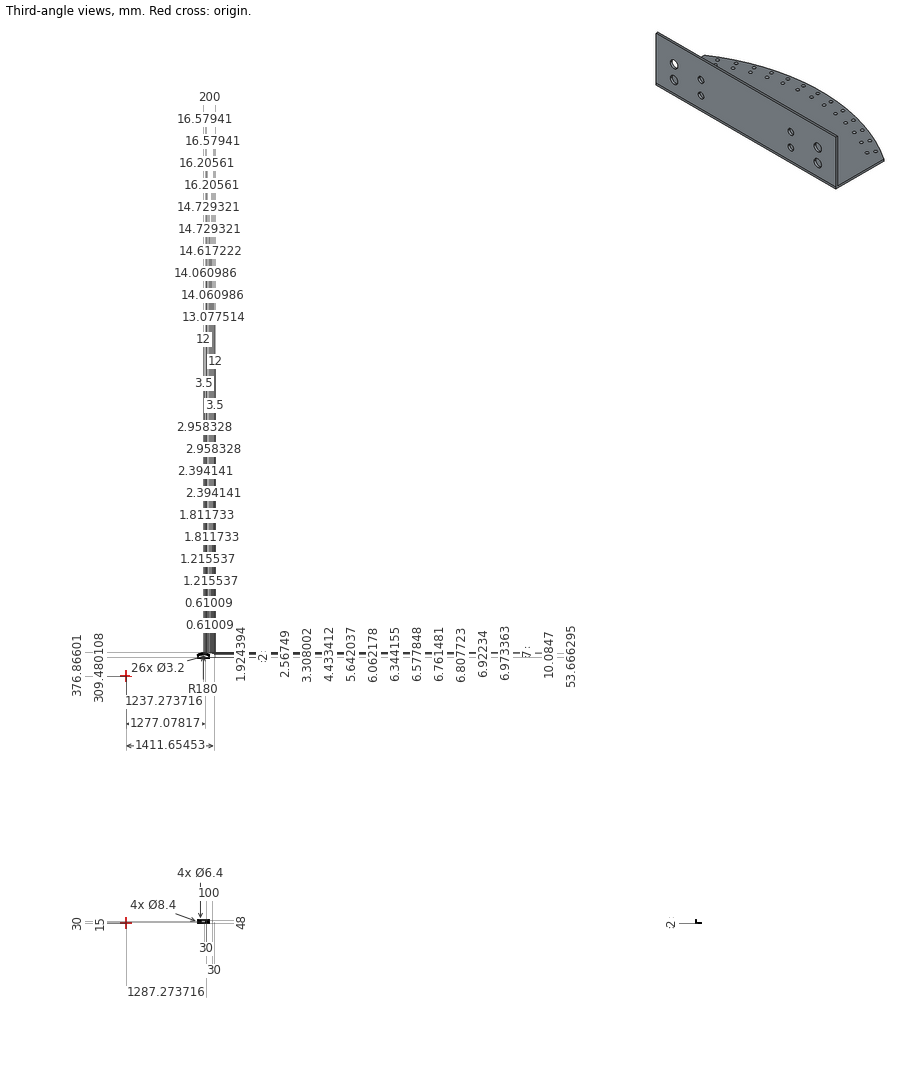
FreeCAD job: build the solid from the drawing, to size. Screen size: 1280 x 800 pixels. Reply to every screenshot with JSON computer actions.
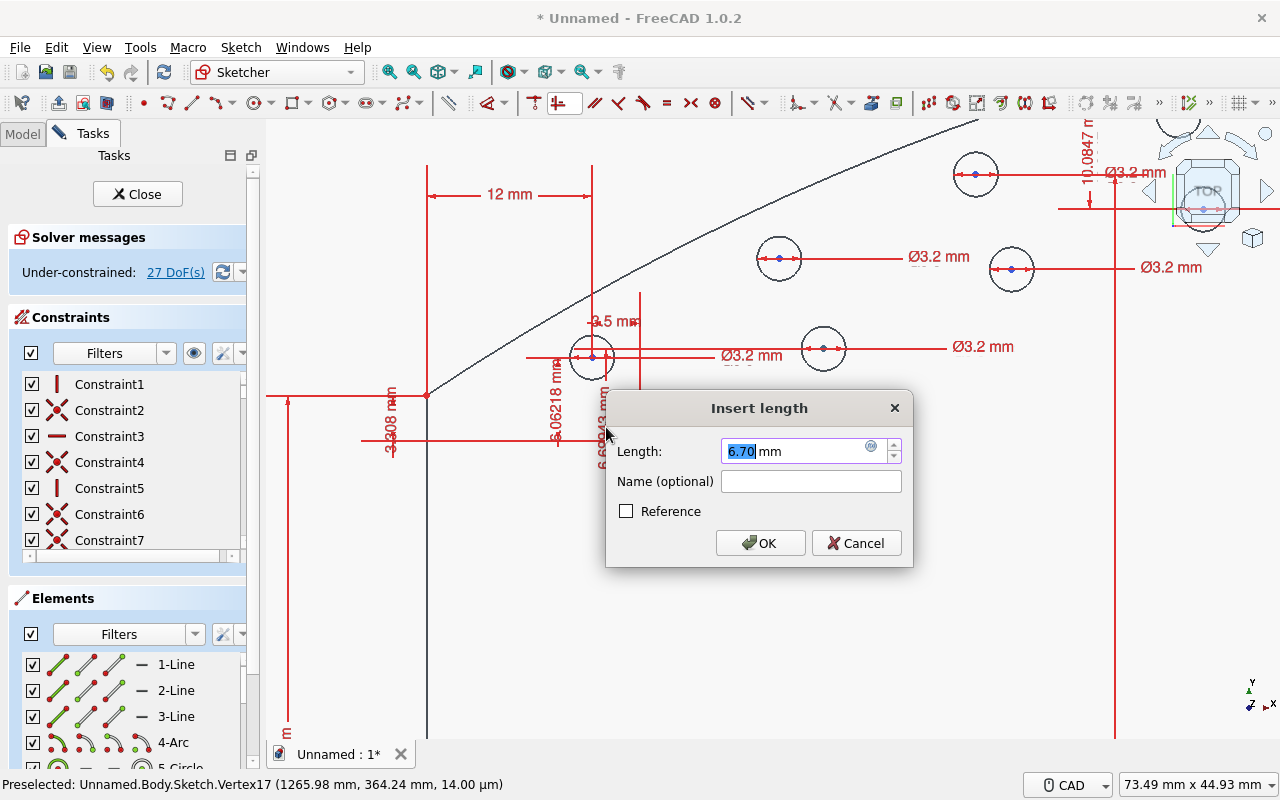
{"action": "type", "text": "6.807723"}
{"action": "key", "text": "Return"}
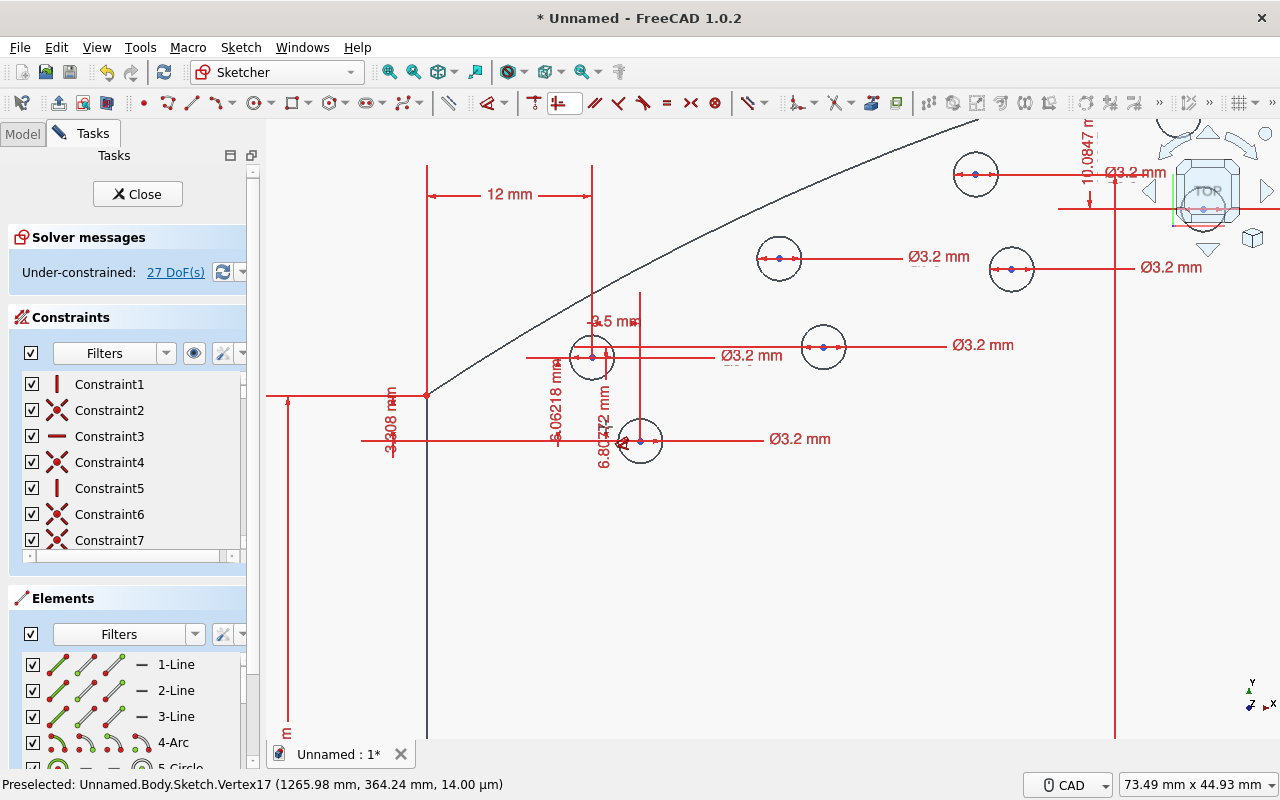
{"action": "left_click", "coordinate": [824, 347]}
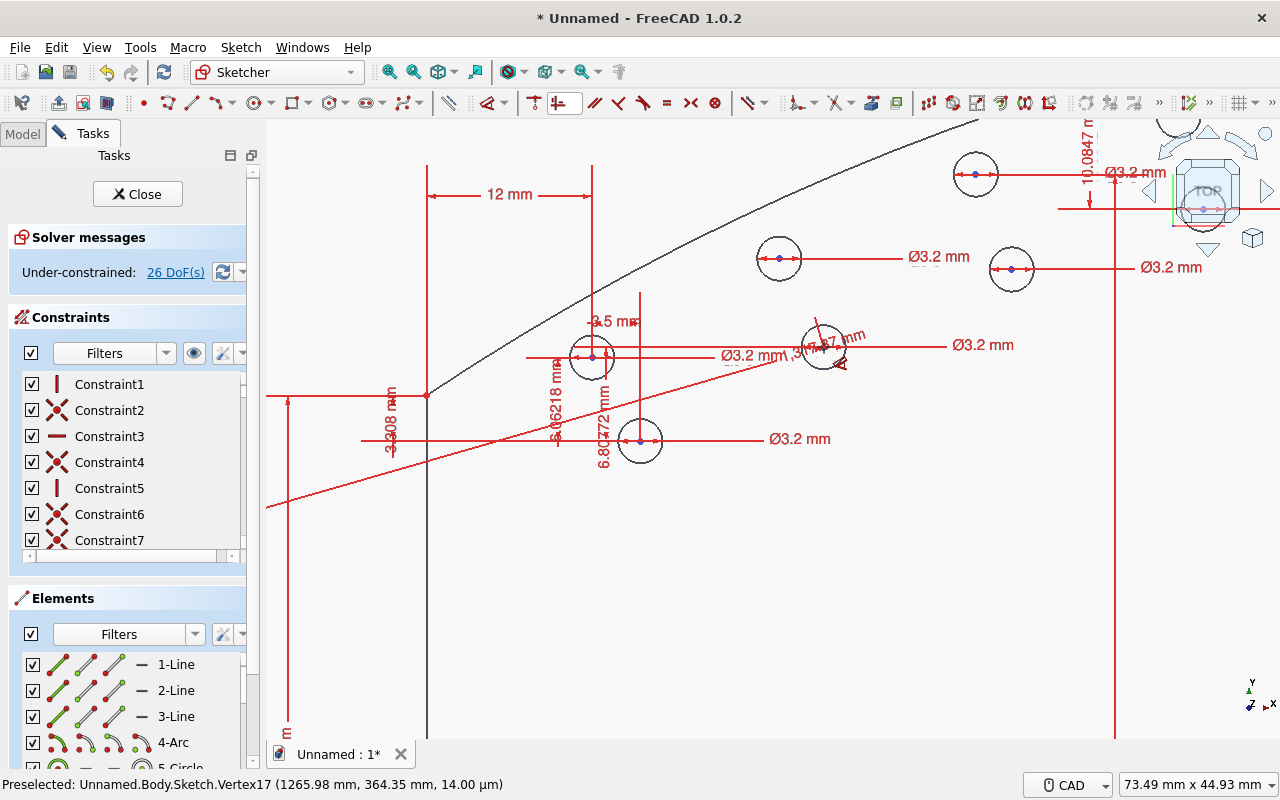
{"action": "left_click", "coordinate": [1012, 269]}
{"action": "left_click", "coordinate": [790, 308]}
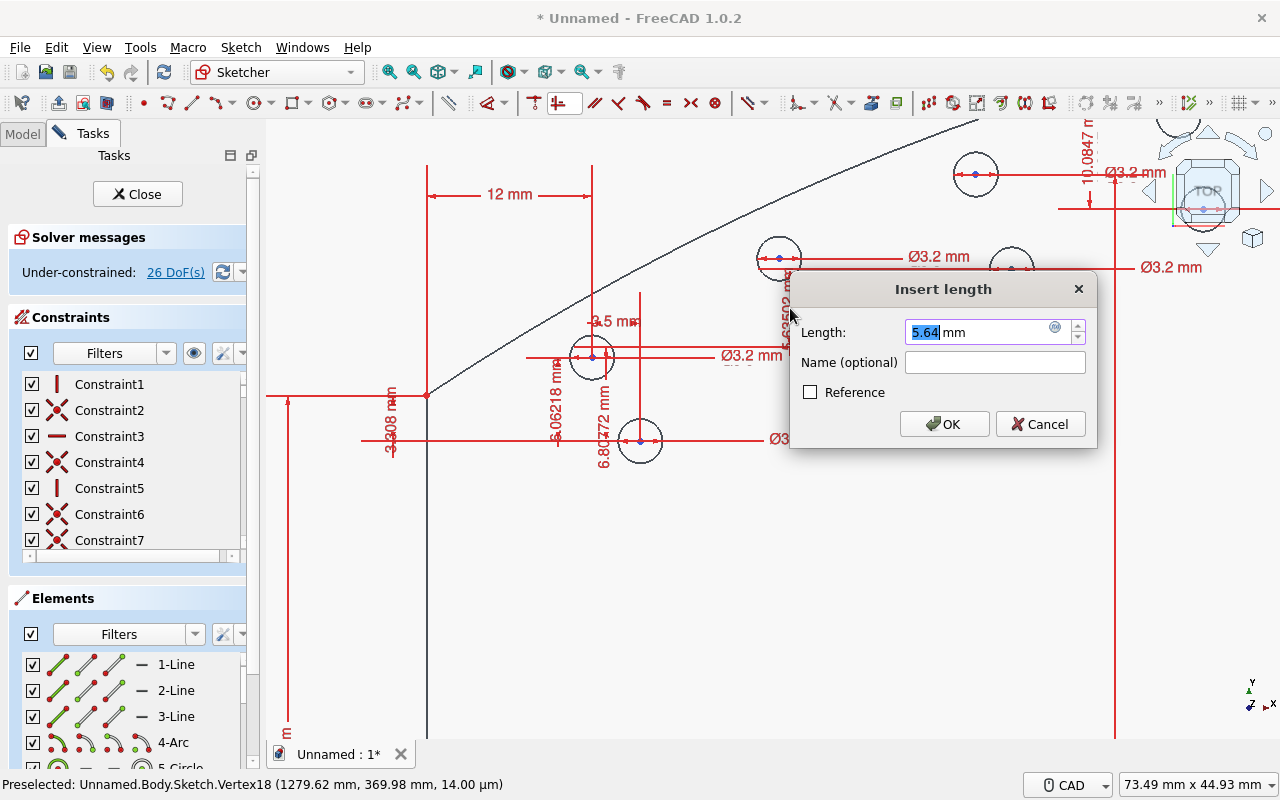
{"action": "type", "text": "5.642037"}
{"action": "key", "text": "Return"}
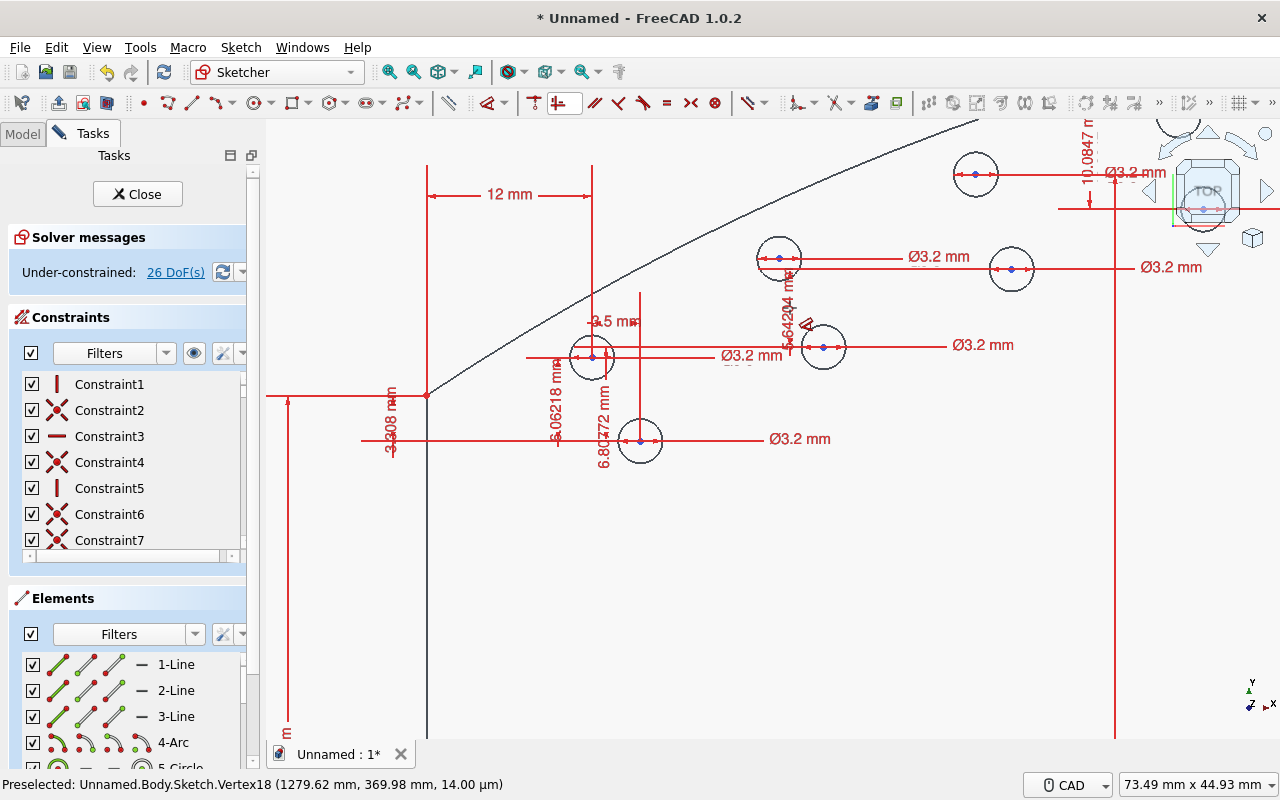
{"action": "left_click", "coordinate": [824, 347]}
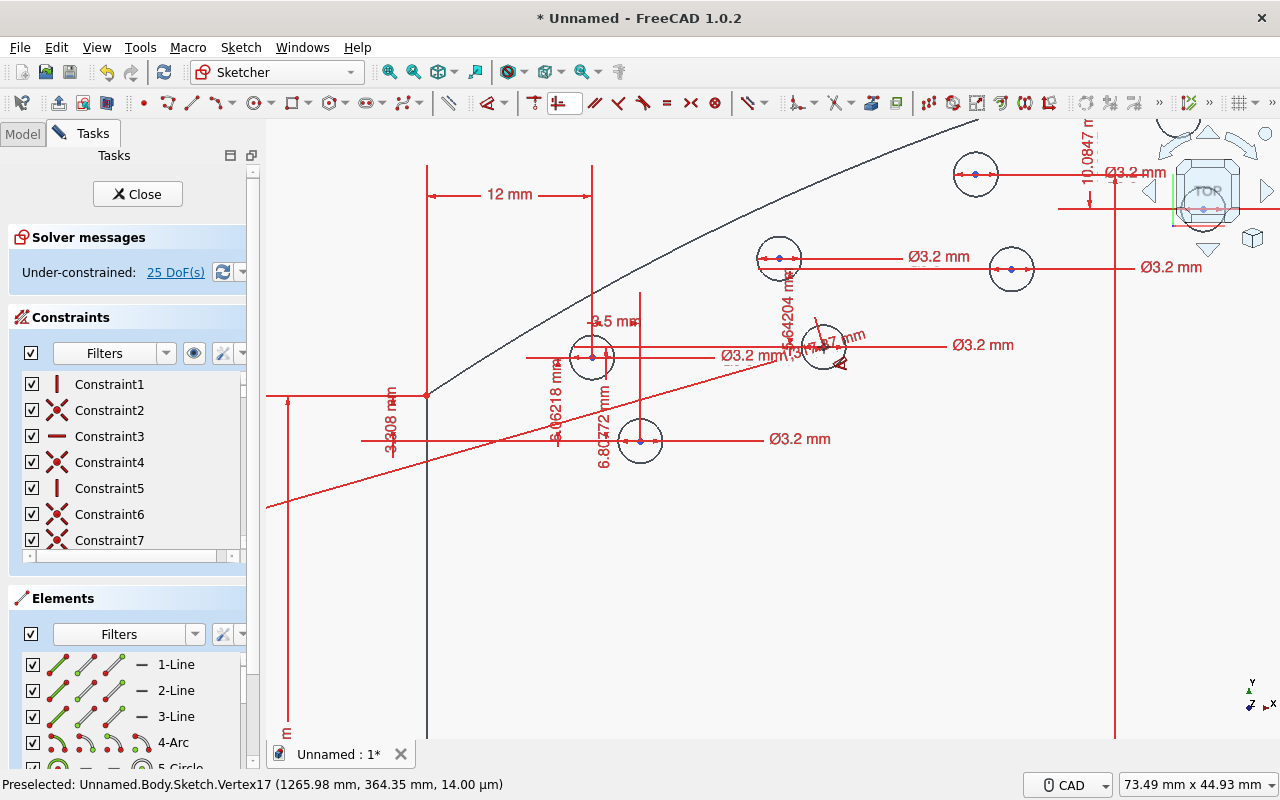
{"action": "left_click", "coordinate": [779, 259]}
{"action": "left_click", "coordinate": [801, 225]}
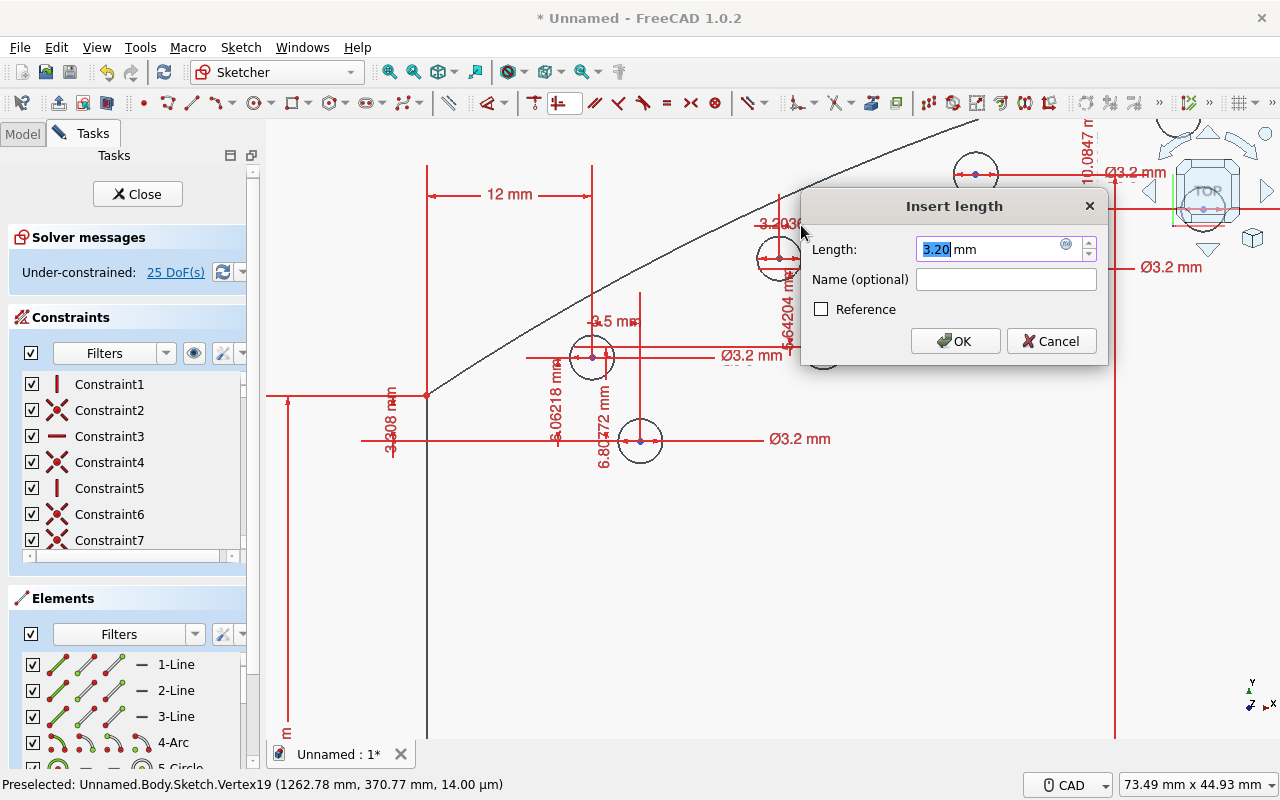
{"action": "type", "text": "2.958328"}
{"action": "key", "text": "Return"}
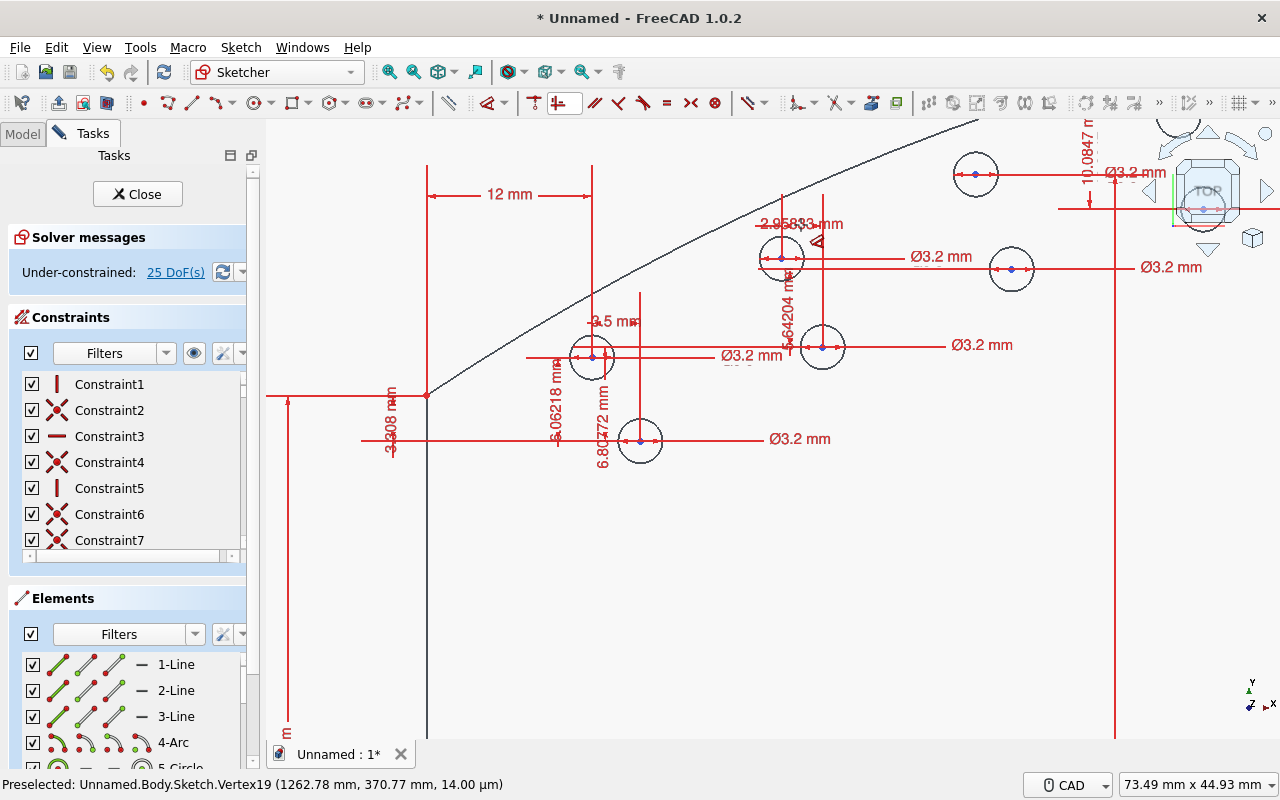
{"action": "scroll", "coordinate": [426, 398], "scroll_direction": "down", "scroll_amount": 8}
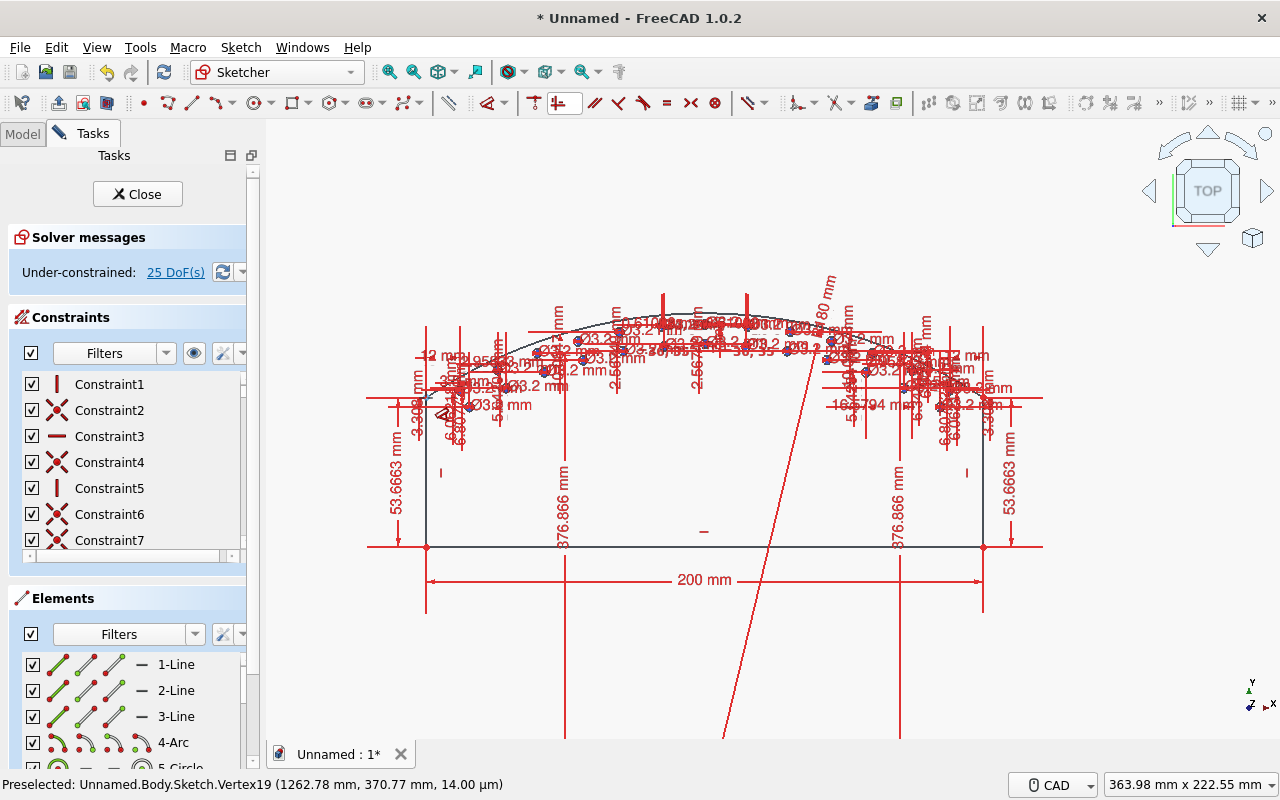
{"action": "left_click", "coordinate": [544, 372]}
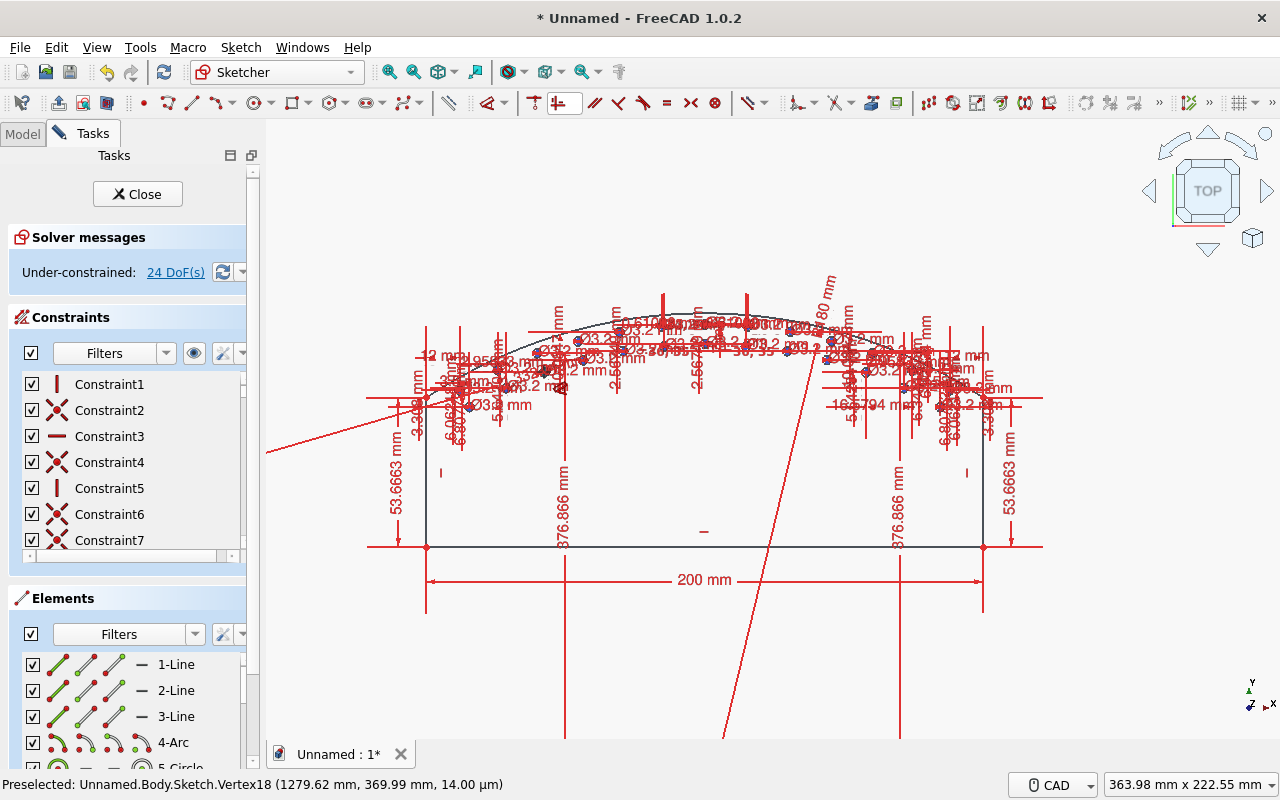
{"action": "left_click", "coordinate": [498, 370]}
{"action": "left_click", "coordinate": [537, 406]}